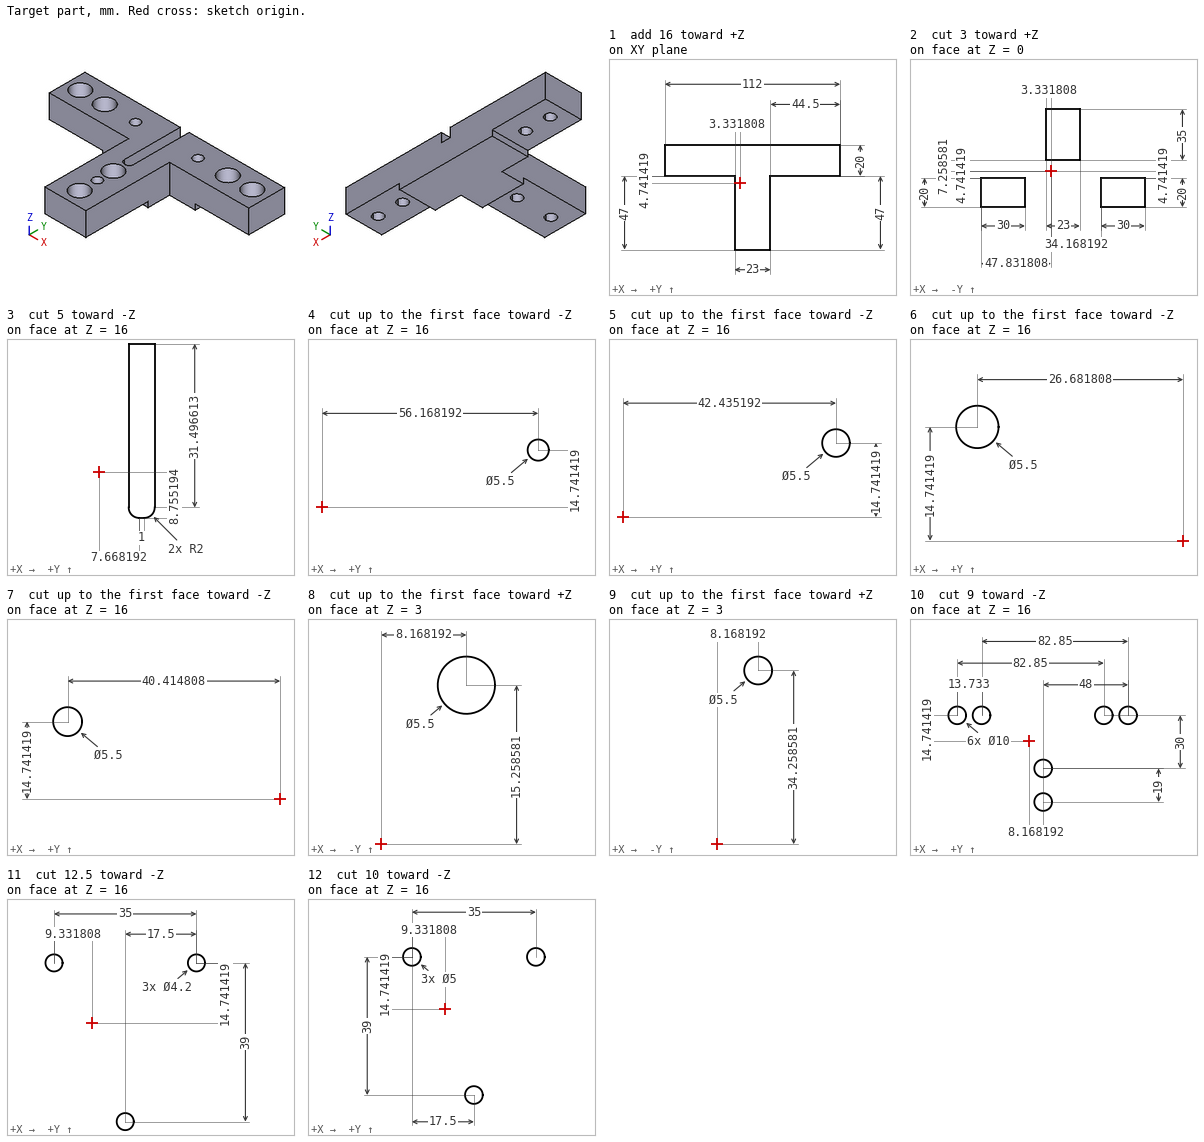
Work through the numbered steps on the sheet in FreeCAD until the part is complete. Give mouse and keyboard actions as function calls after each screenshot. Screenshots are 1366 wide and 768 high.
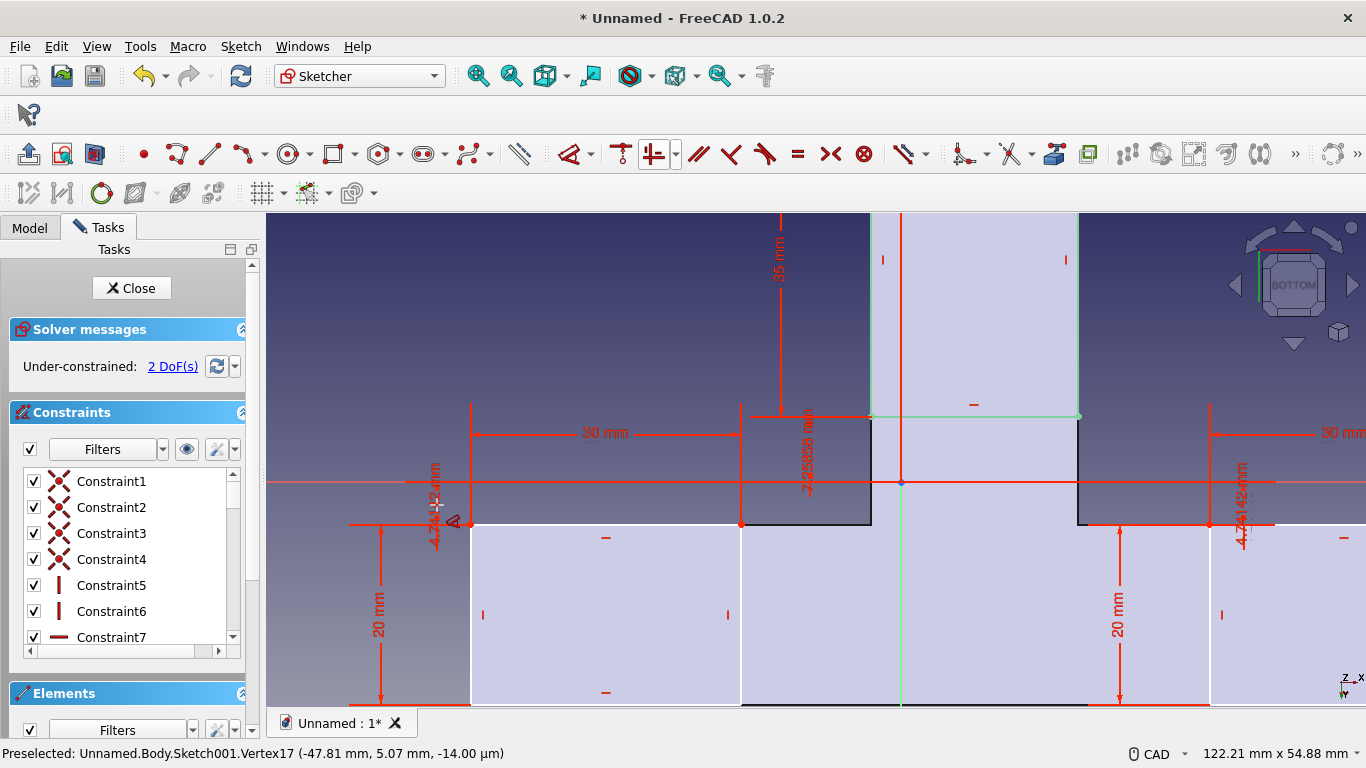
scroll(471, 529, down, 3)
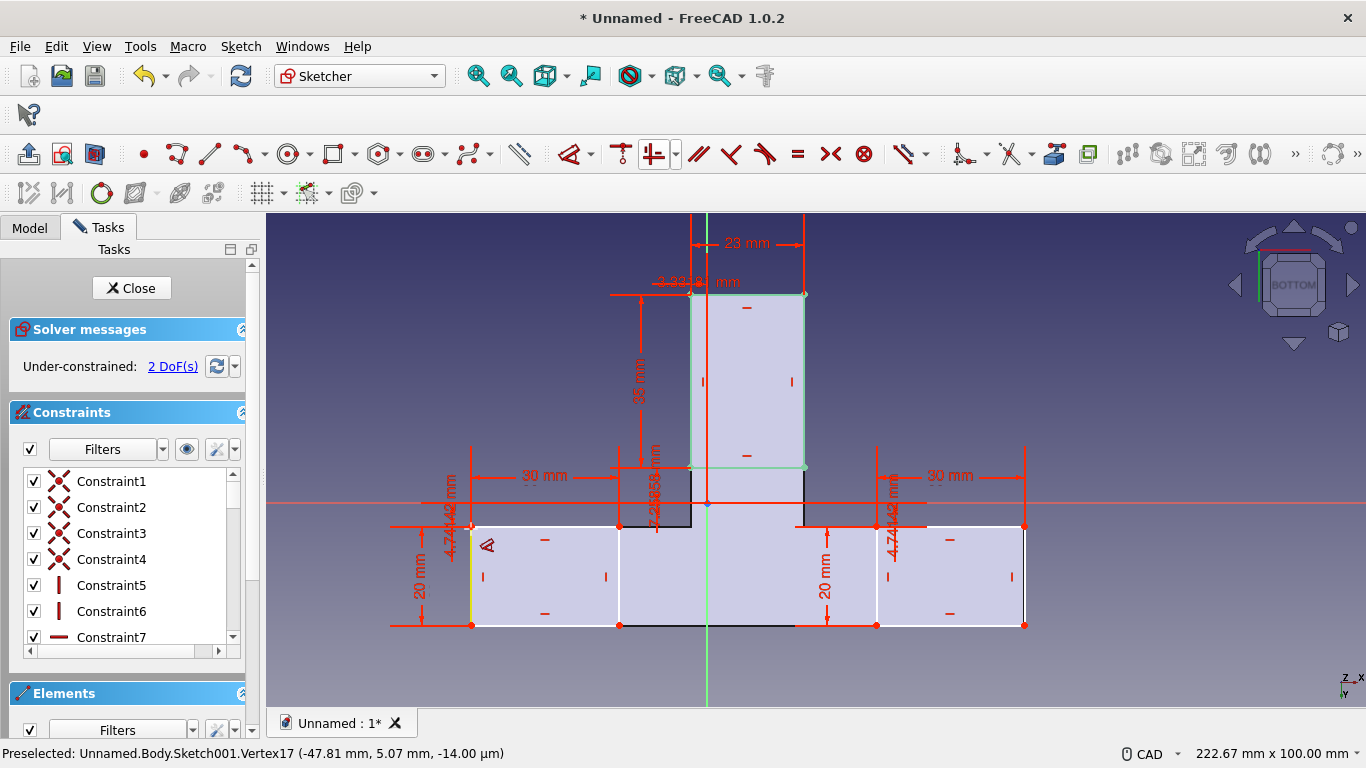
click(877, 527)
click(792, 561)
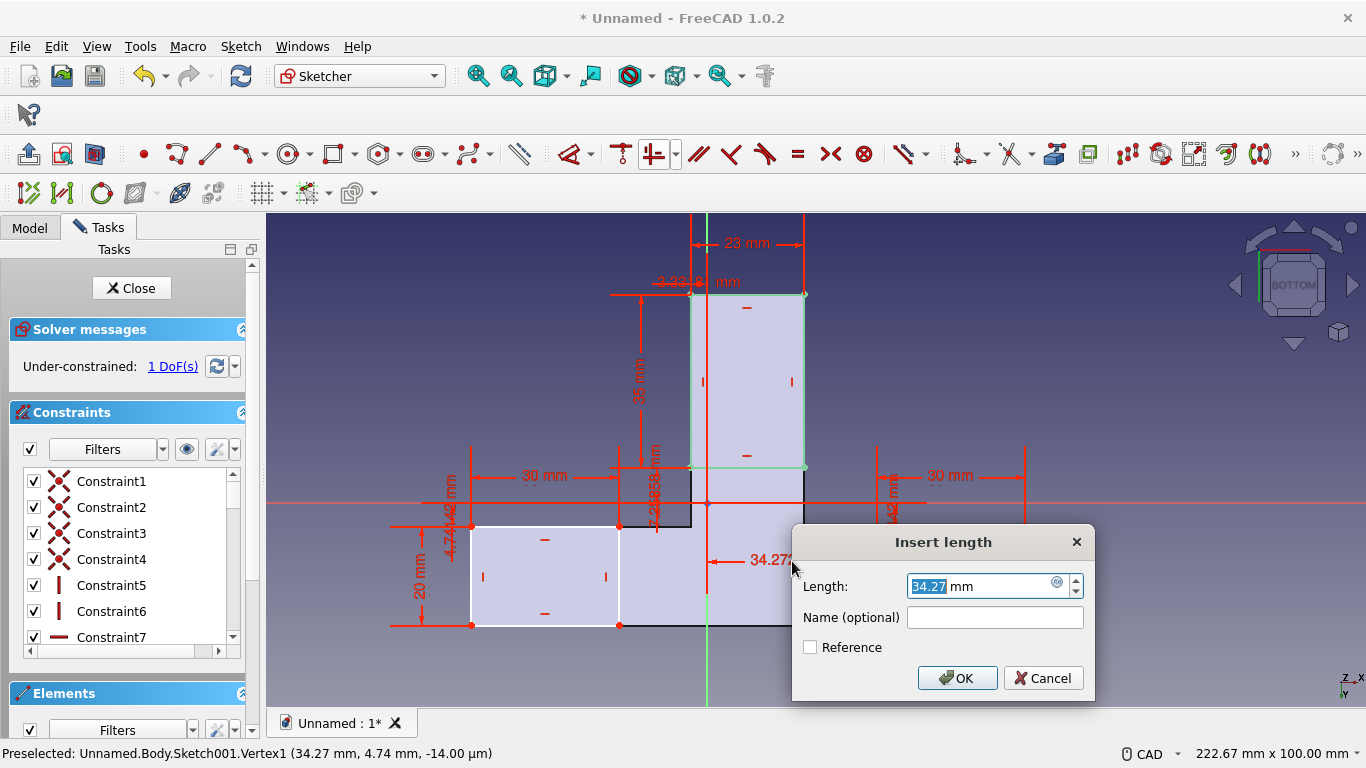
text(34.168192)
key(Return)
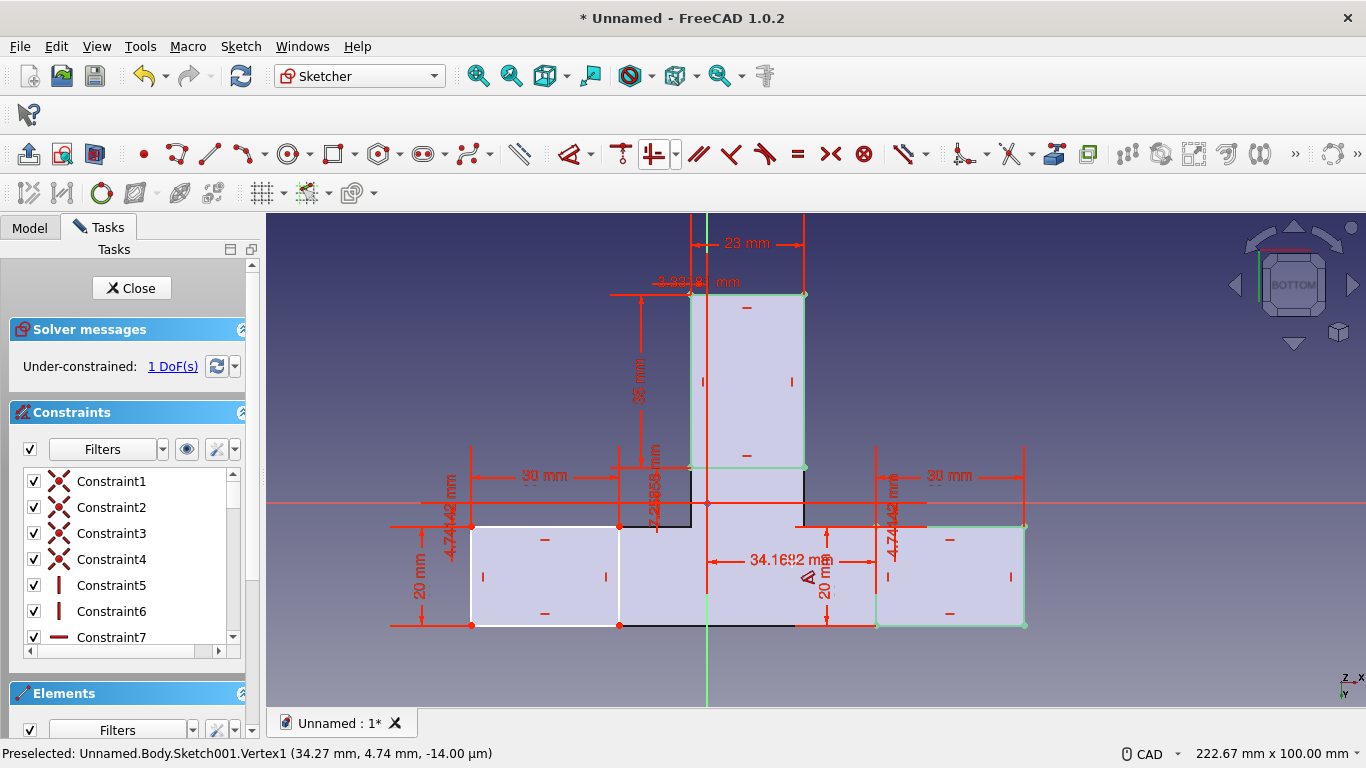
click(471, 527)
click(589, 561)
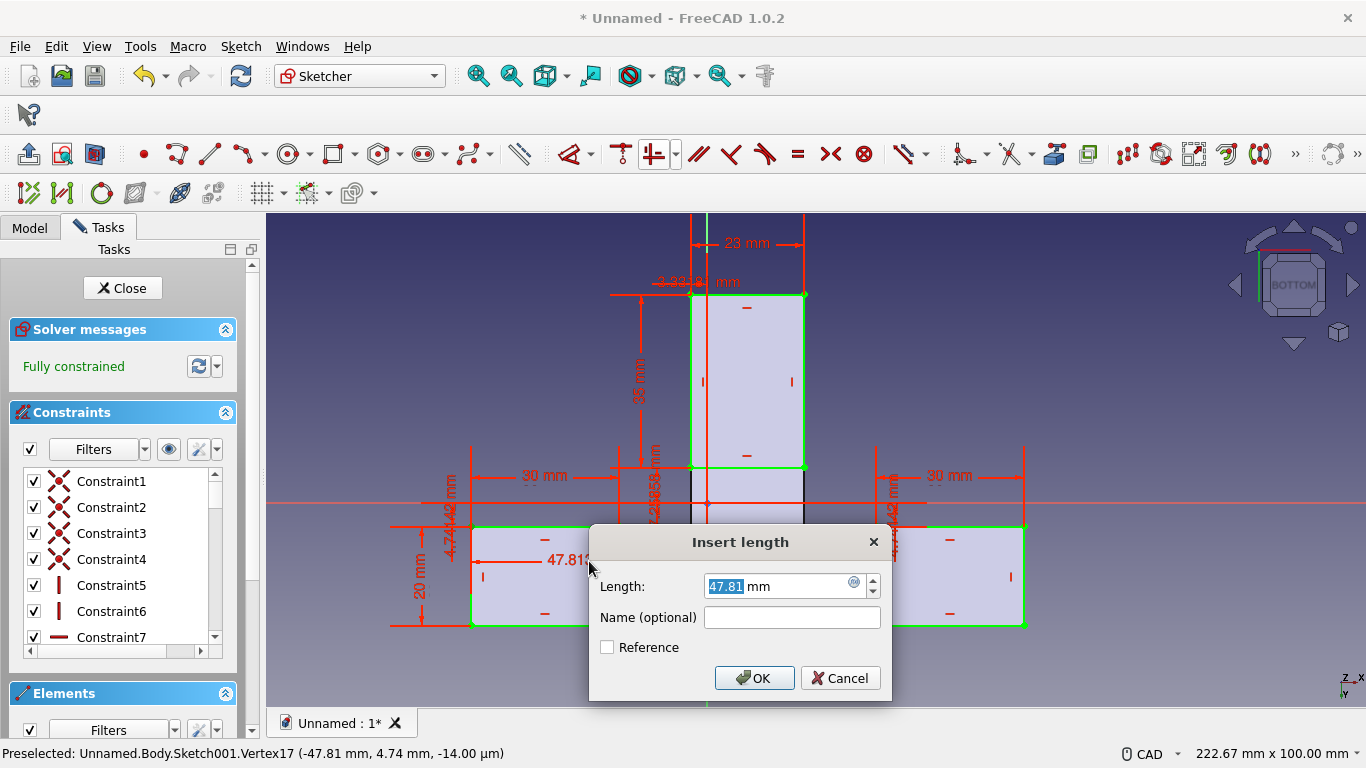
text(47.831808)
key(Return)
key(Escape)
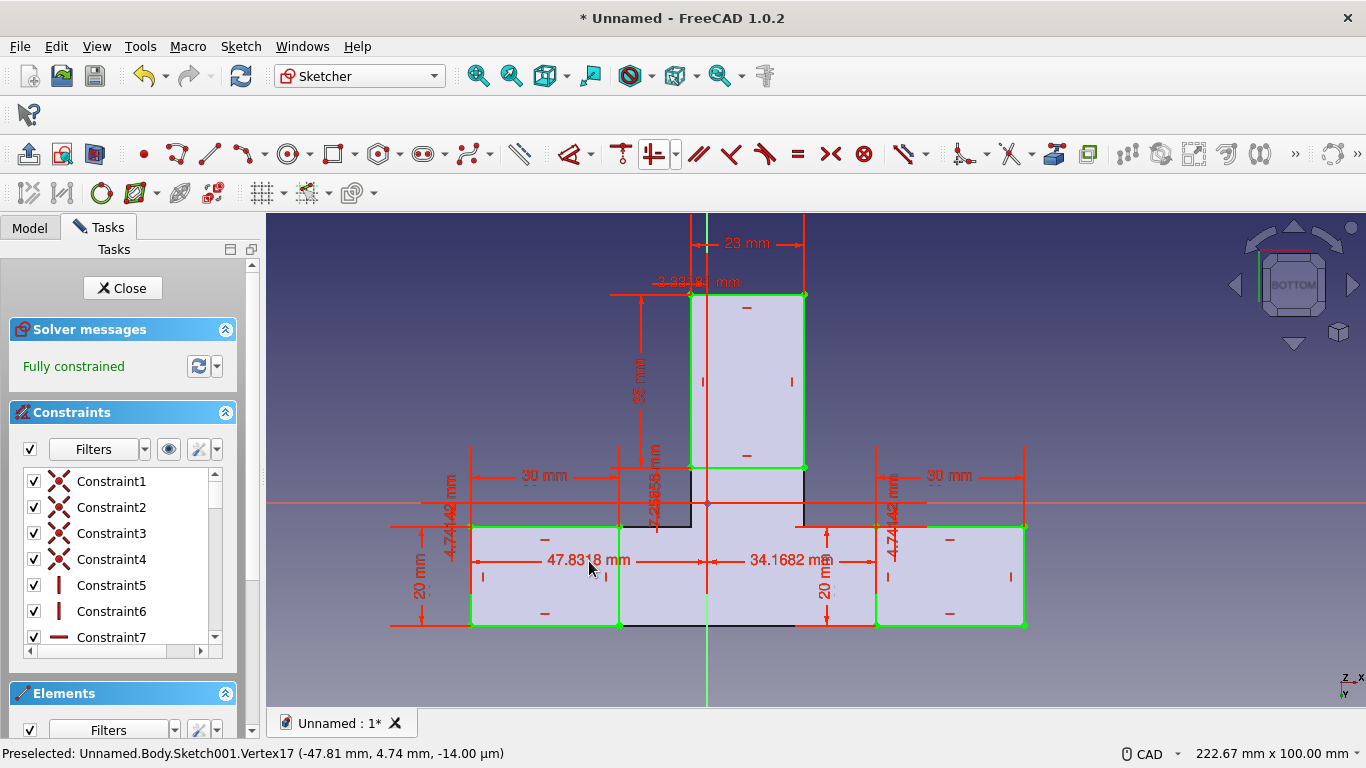
click(123, 288)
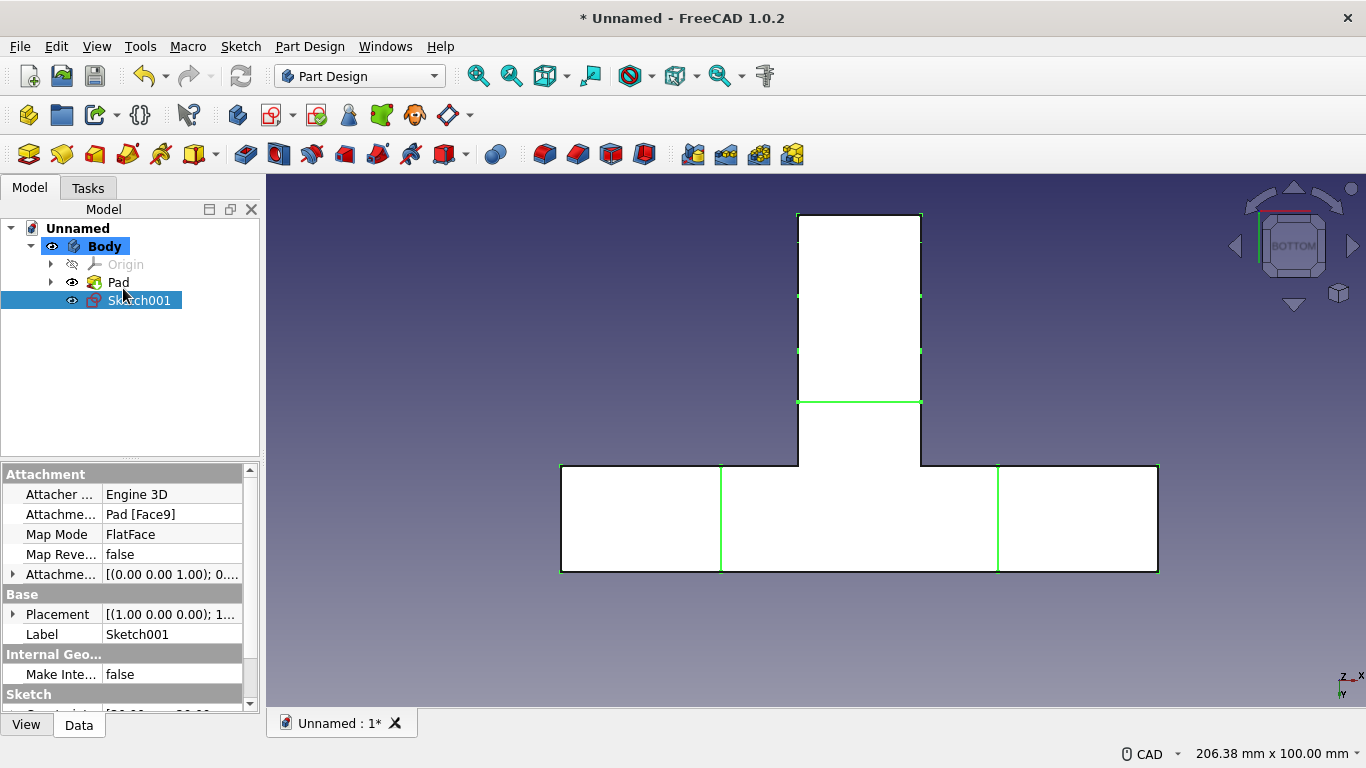
click(246, 154)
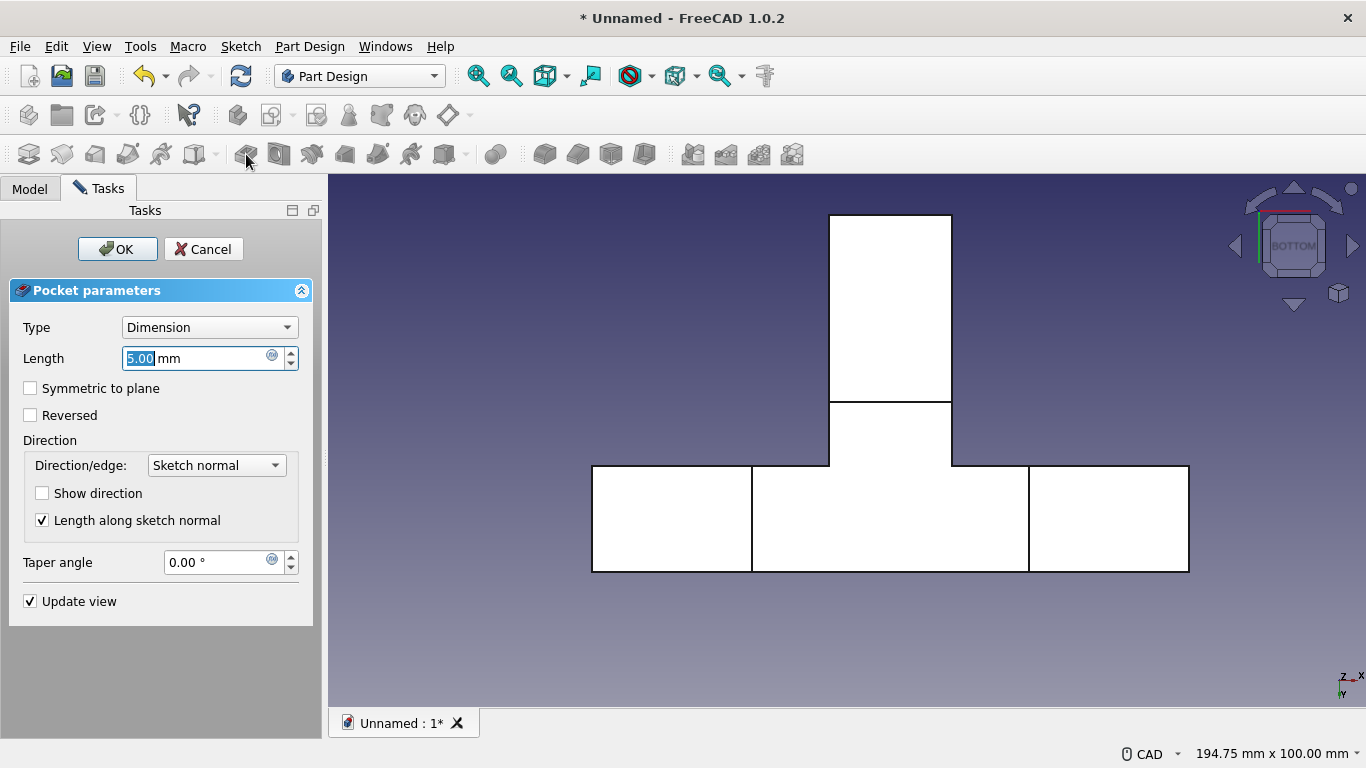
text(3)
key(Tab)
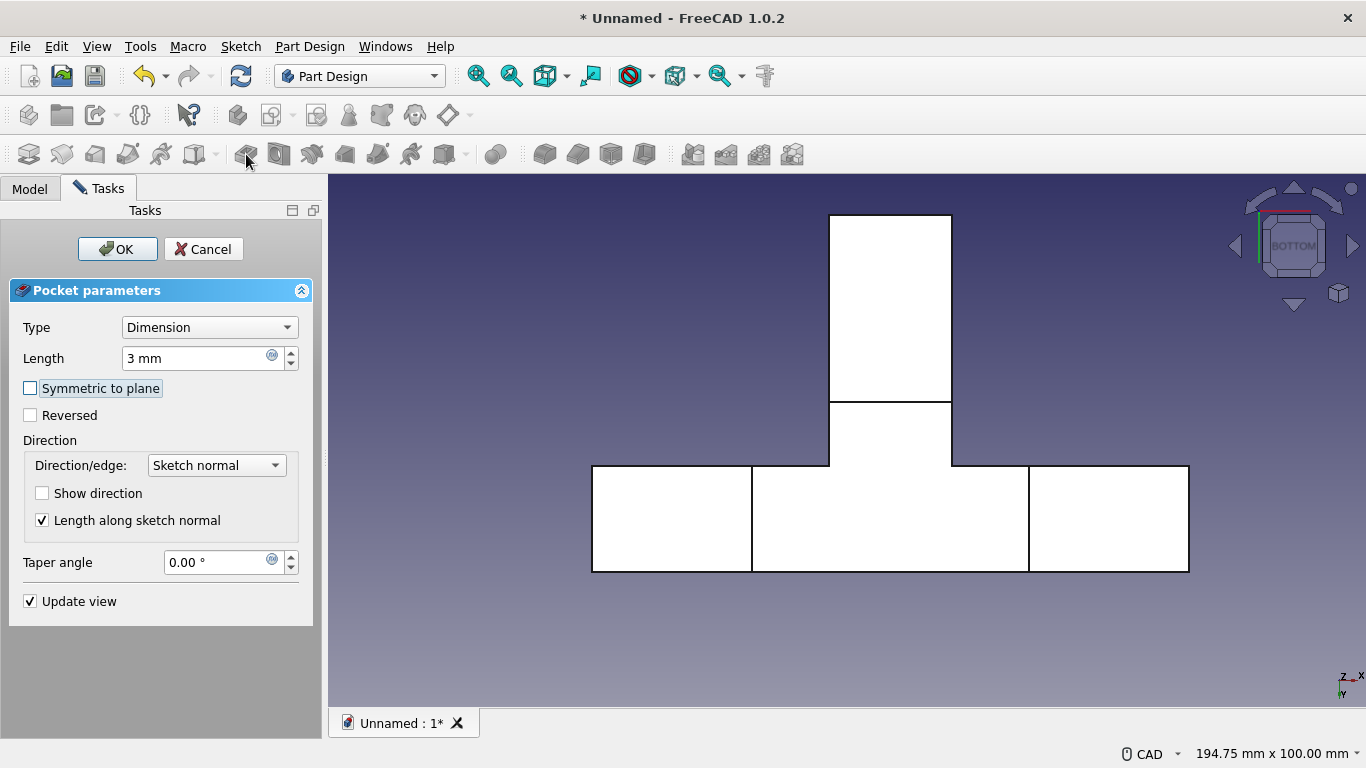
click(118, 249)